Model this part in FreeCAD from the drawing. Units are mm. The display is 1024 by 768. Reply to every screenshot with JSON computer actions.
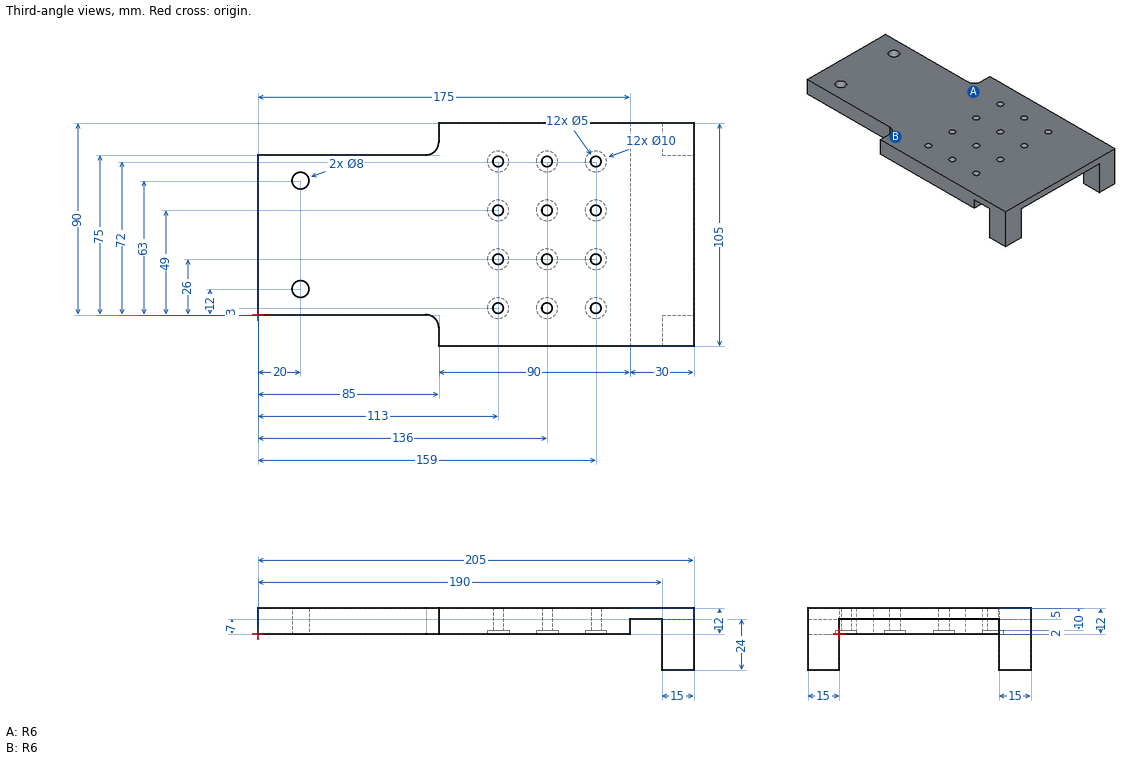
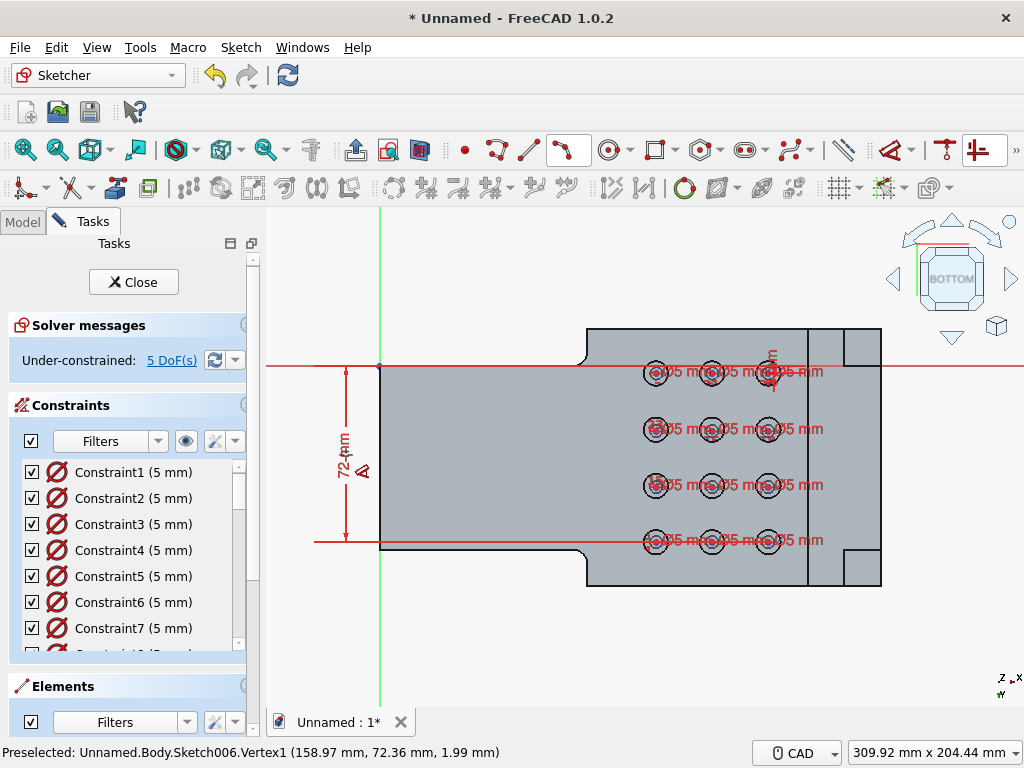
{"action": "left_click", "coordinate": [656, 487]}
{"action": "left_click", "coordinate": [346, 427]}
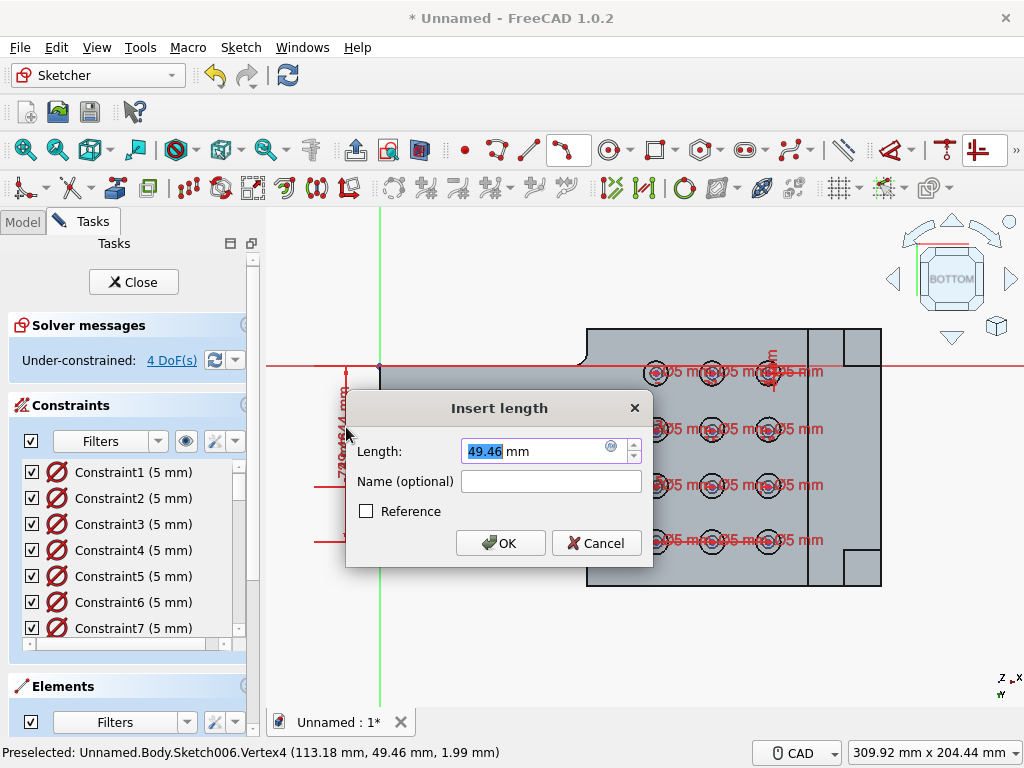
{"action": "type", "text": "49"}
{"action": "key", "text": "Return"}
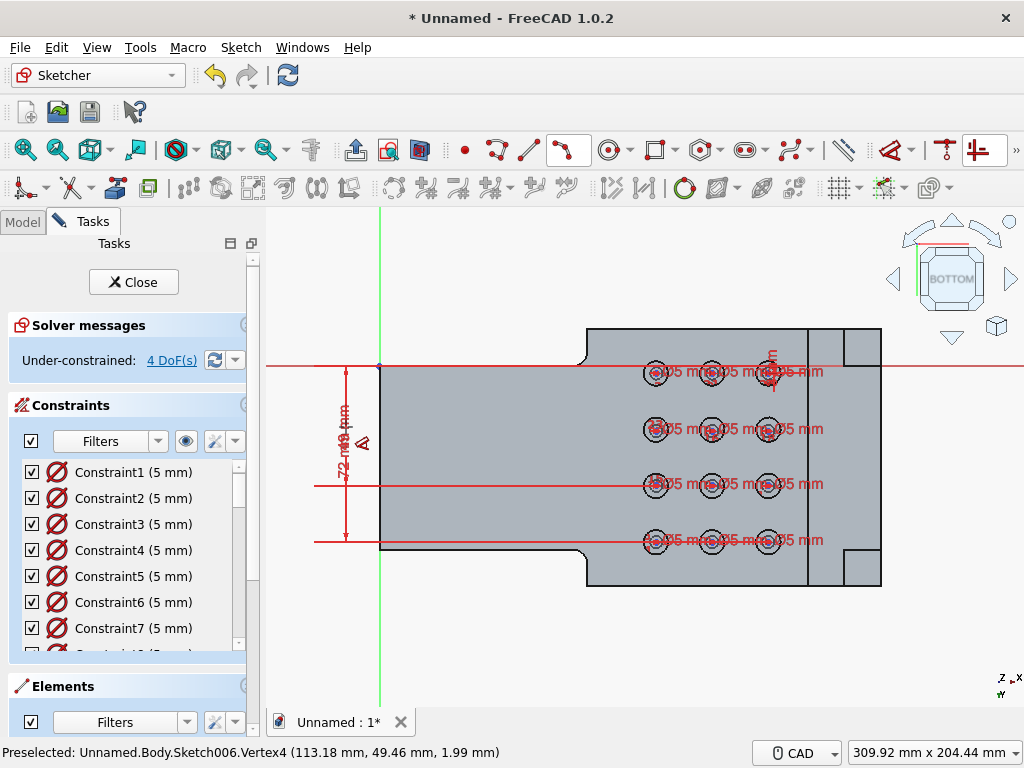
{"action": "left_click", "coordinate": [768, 431]}
{"action": "left_click", "coordinate": [346, 399]}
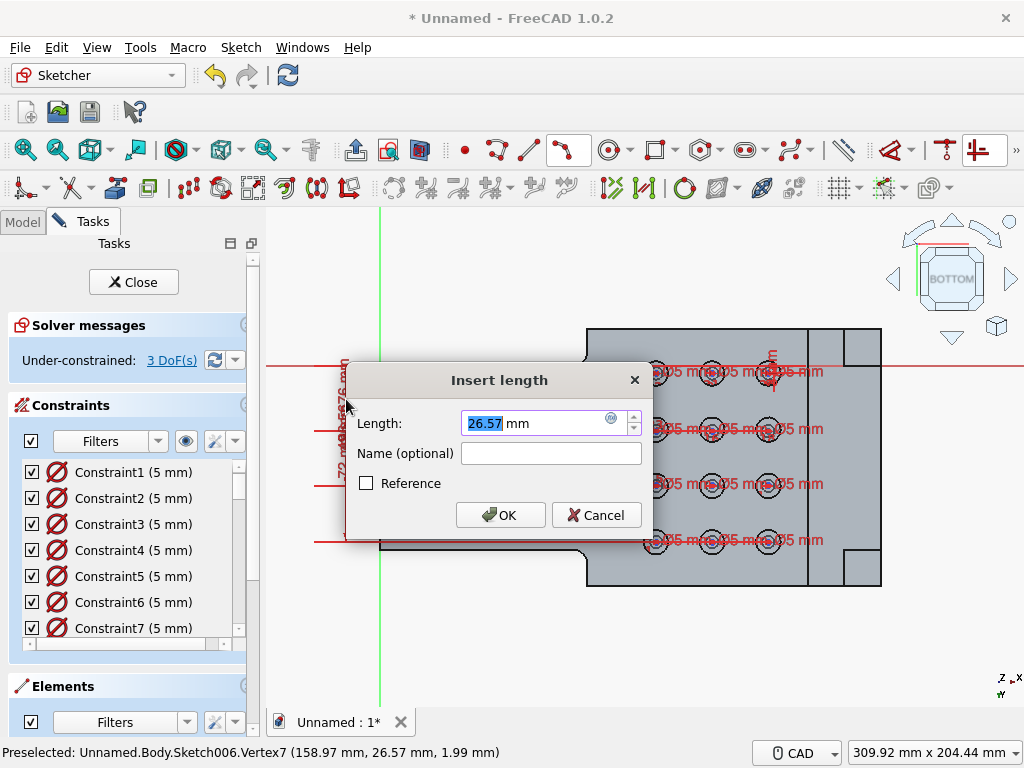
{"action": "type", "text": "26"}
{"action": "key", "text": "Return"}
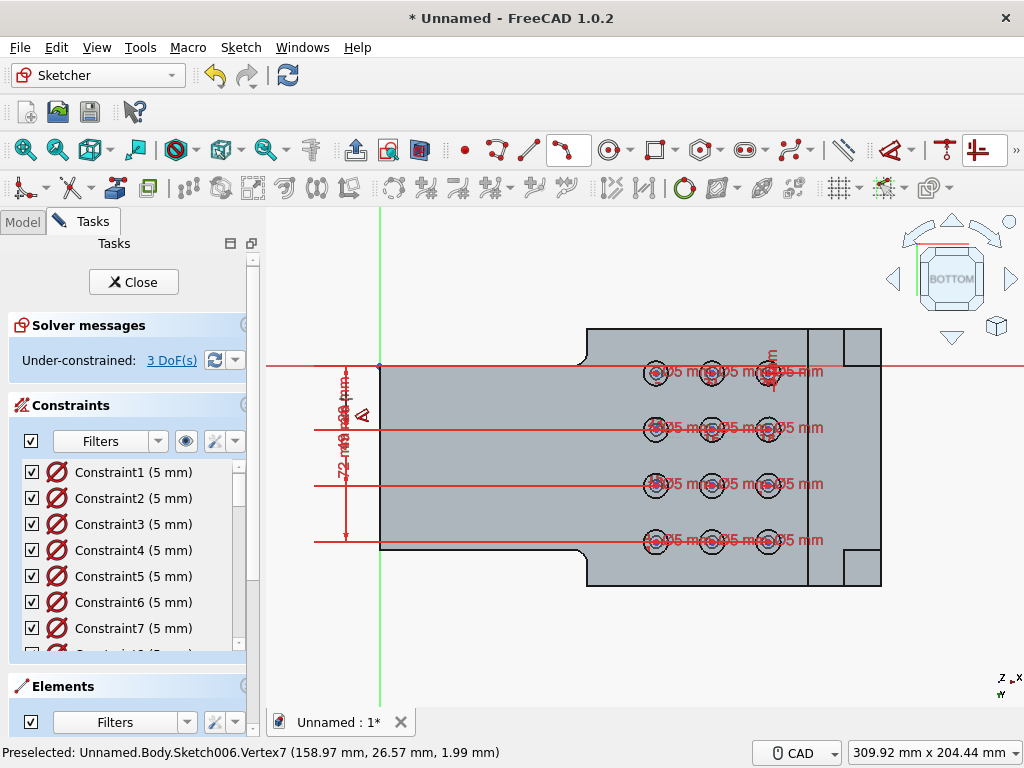
{"action": "left_click", "coordinate": [768, 542]}
{"action": "left_click", "coordinate": [574, 332]}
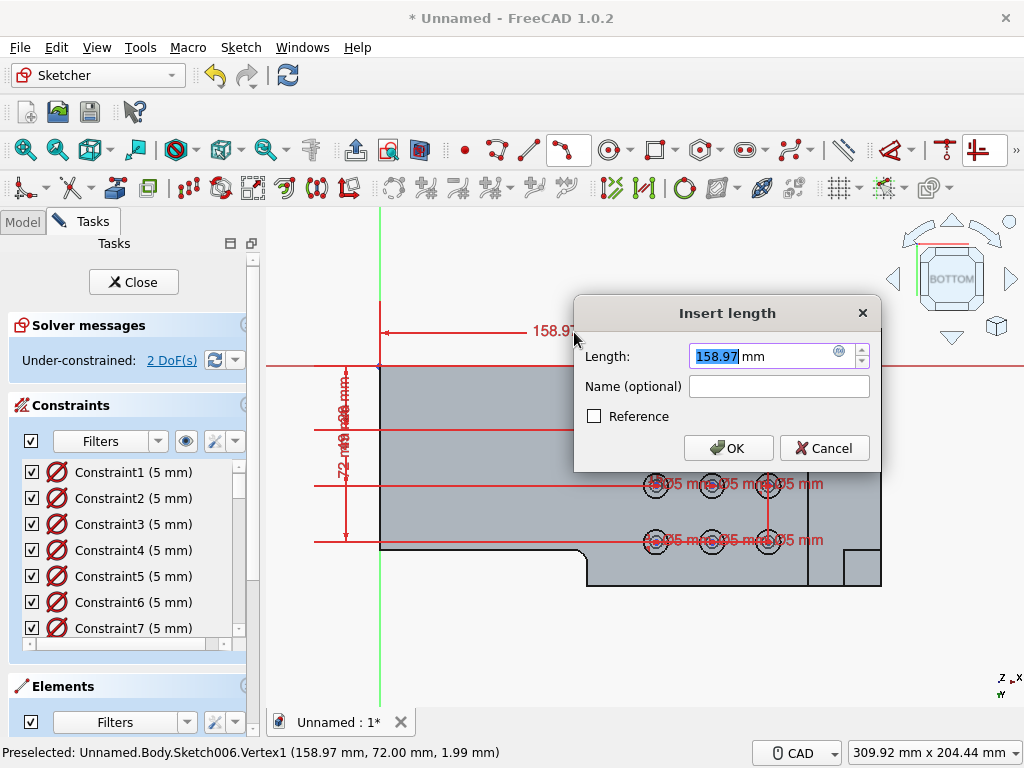
{"action": "type", "text": "159"}
{"action": "key", "text": "Return"}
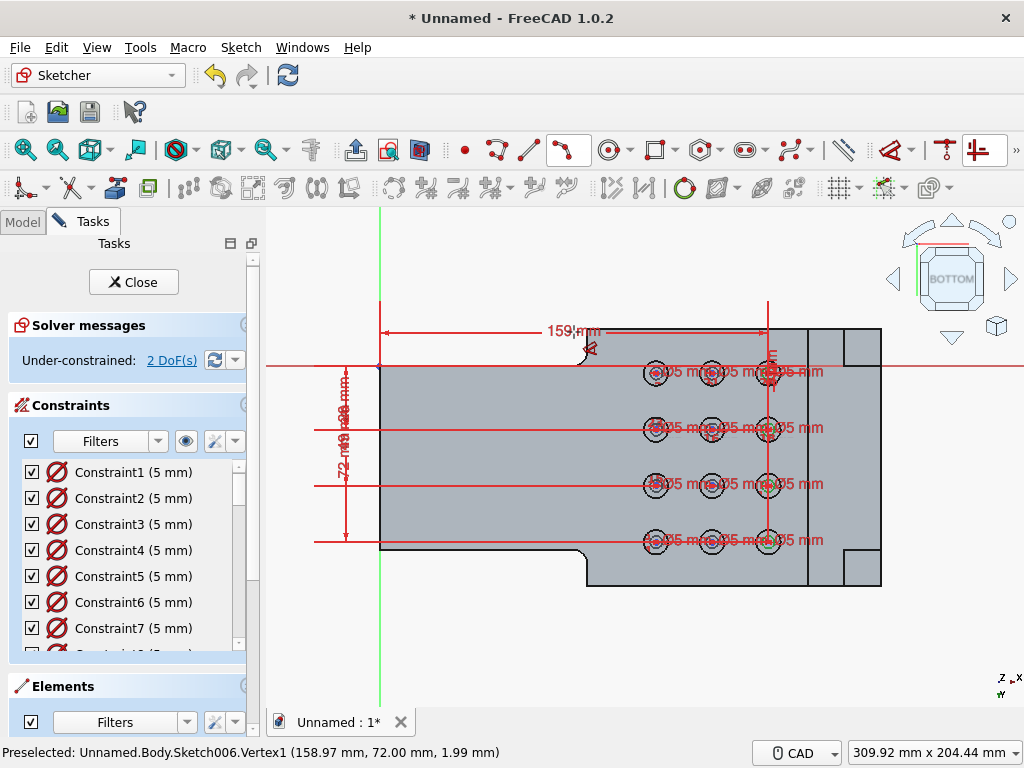
{"action": "left_click", "coordinate": [712, 542]}
{"action": "left_click", "coordinate": [469, 332]}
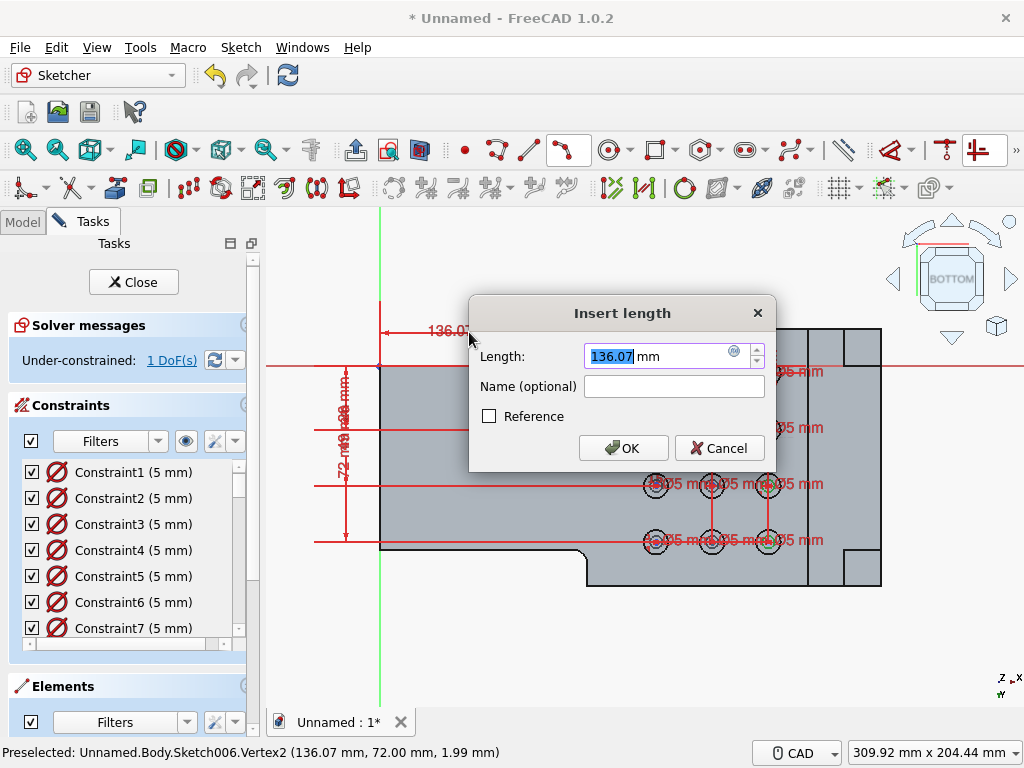
{"action": "type", "text": "136"}
{"action": "key", "text": "Return"}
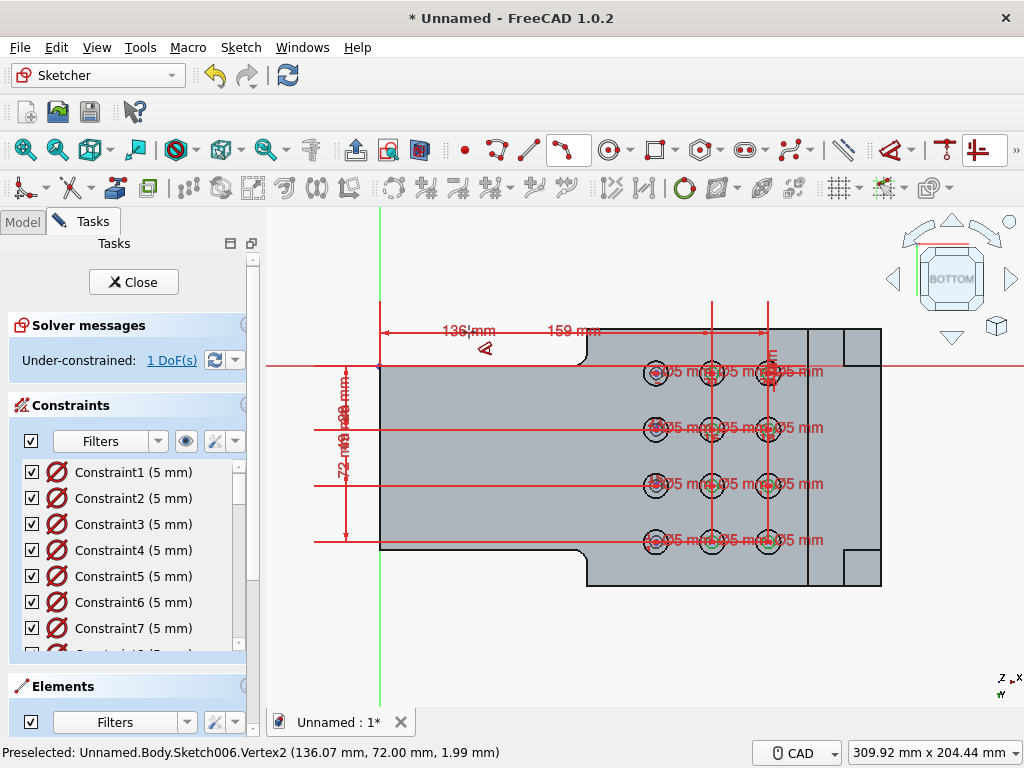
{"action": "left_click", "coordinate": [656, 542]}
{"action": "left_click", "coordinate": [518, 576]}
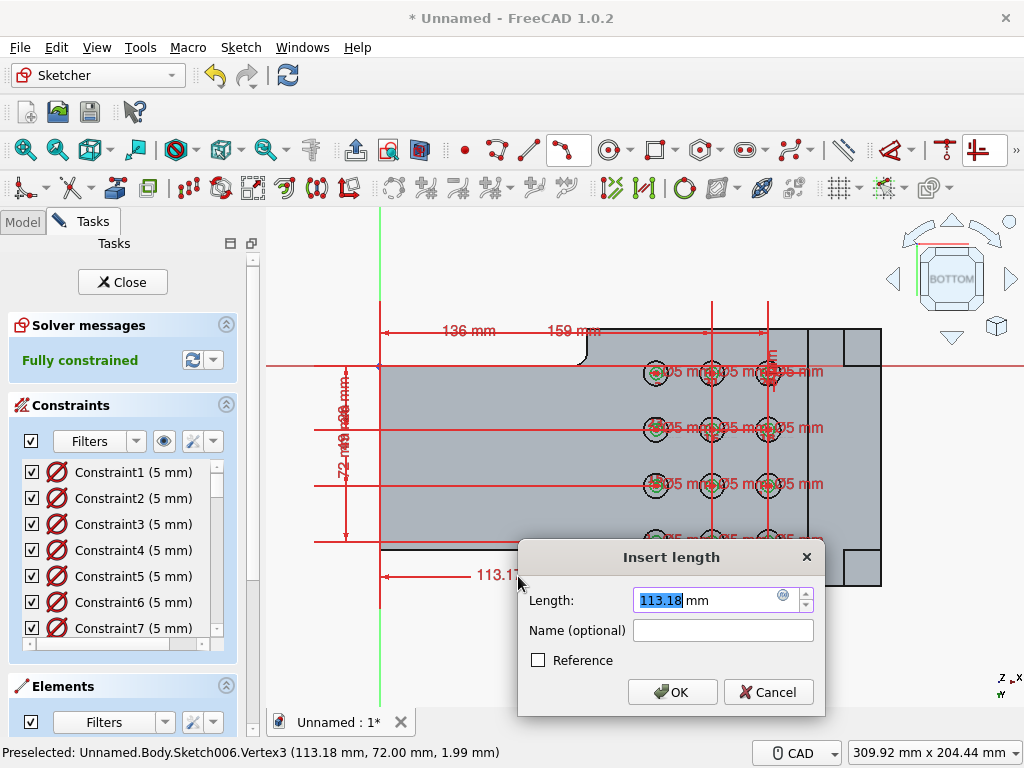
{"action": "type", "text": "113"}
{"action": "key", "text": "Return"}
{"action": "key", "text": "Escape"}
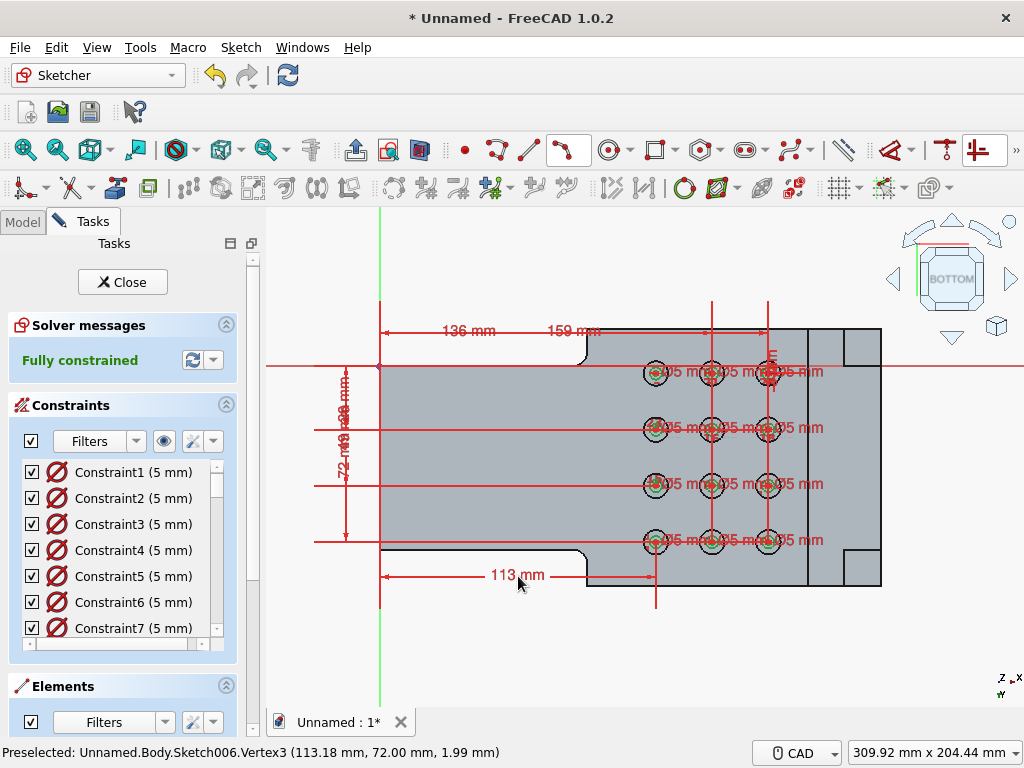
{"action": "left_click", "coordinate": [123, 282]}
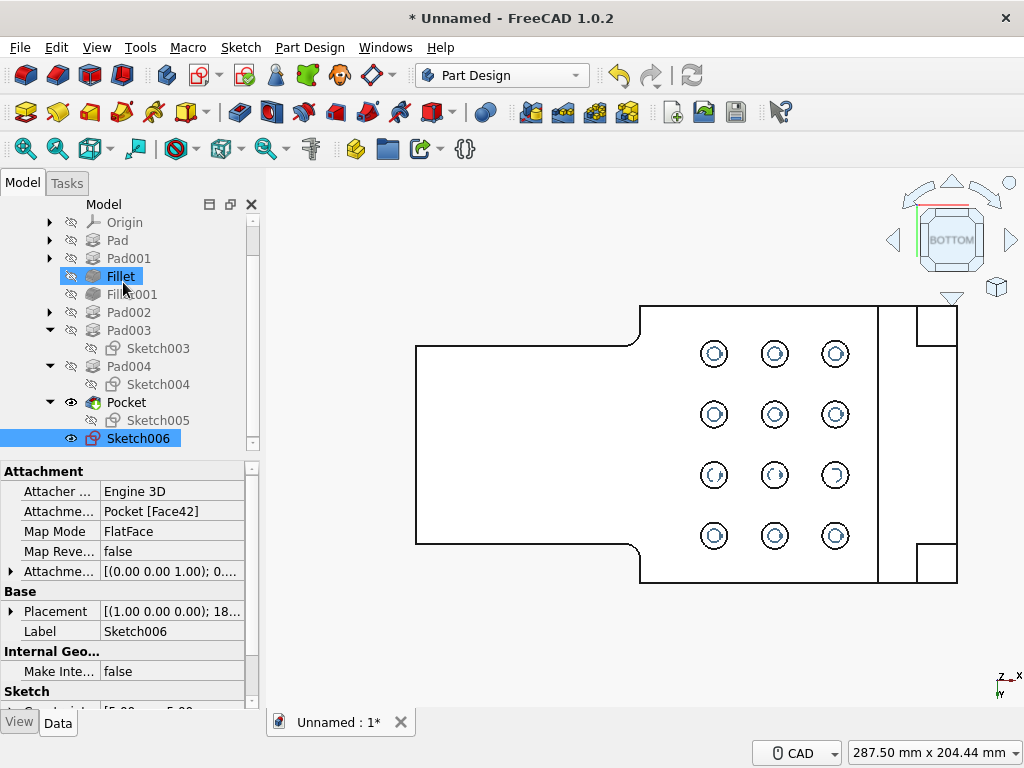
{"action": "left_click", "coordinate": [240, 112]}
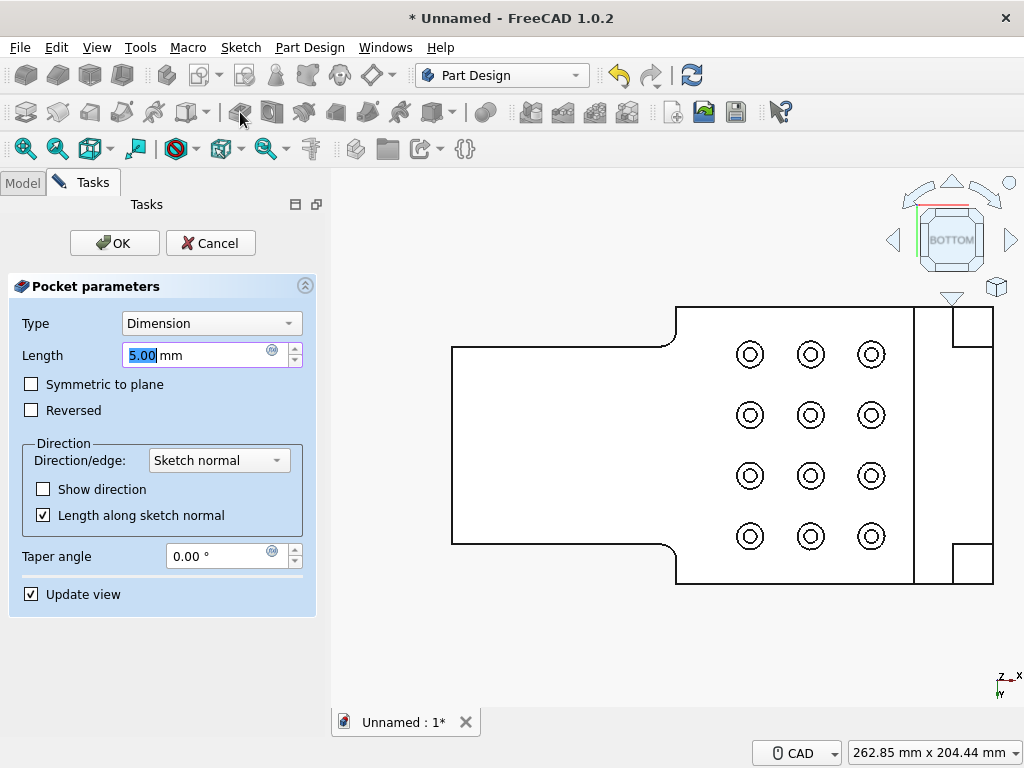
{"action": "type", "text": "10"}
{"action": "key", "text": "Tab"}